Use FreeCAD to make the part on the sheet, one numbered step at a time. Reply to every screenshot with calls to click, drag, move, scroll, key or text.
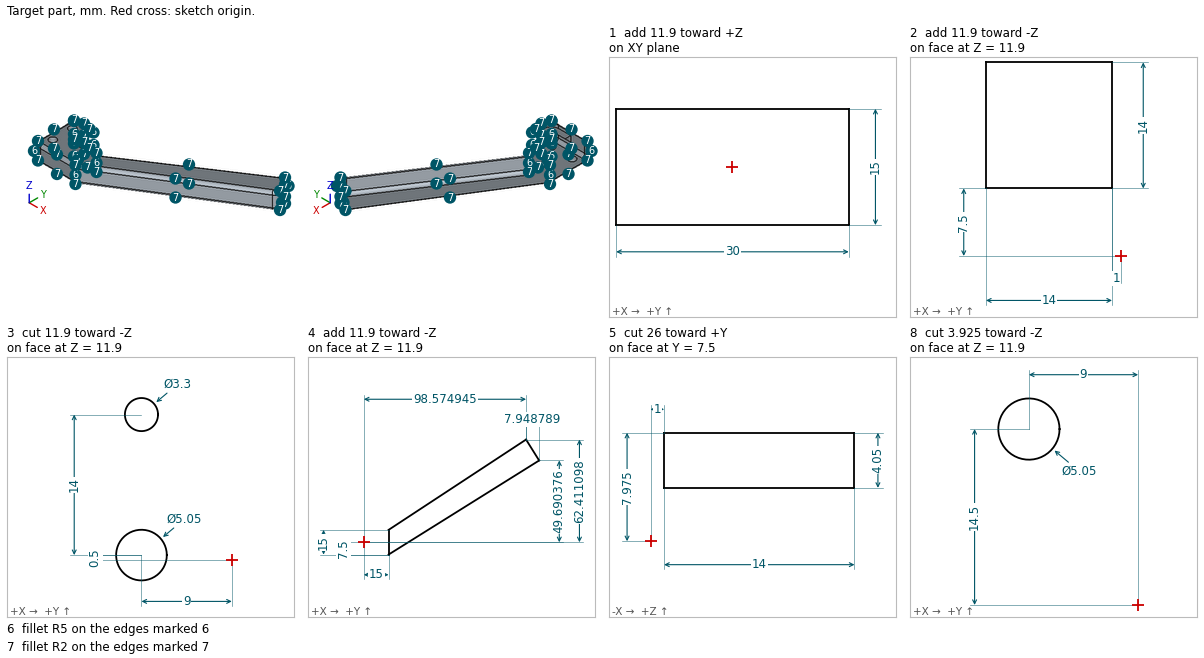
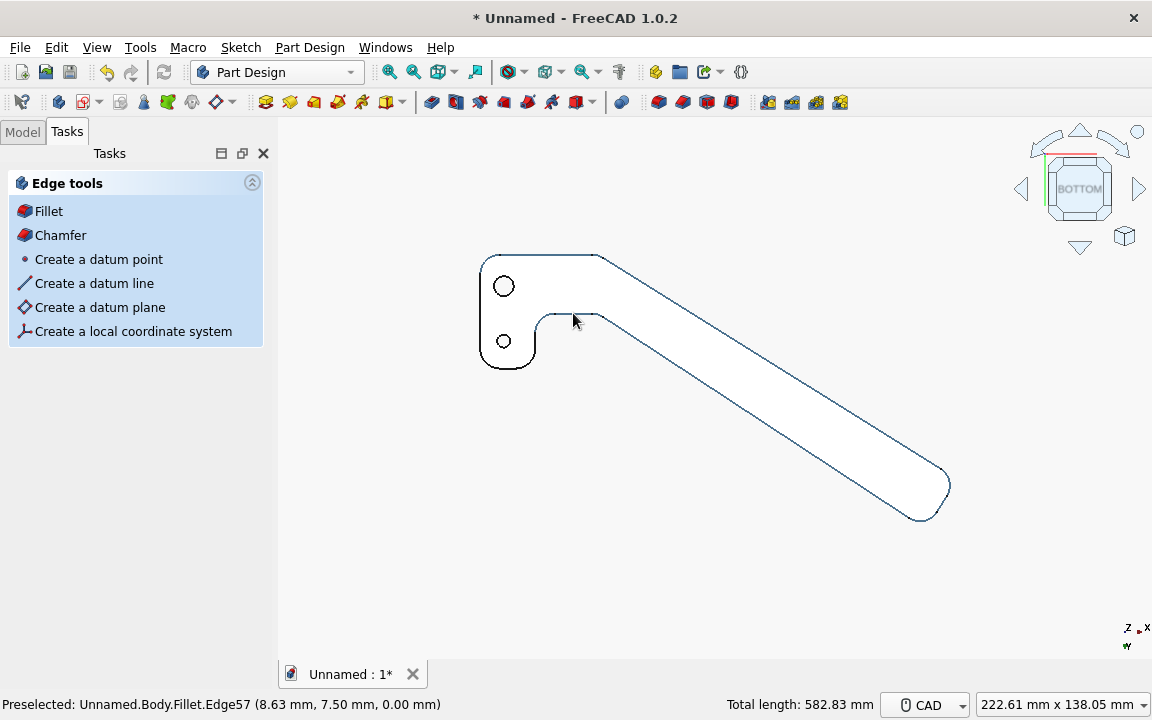
click(480, 349, ctrl)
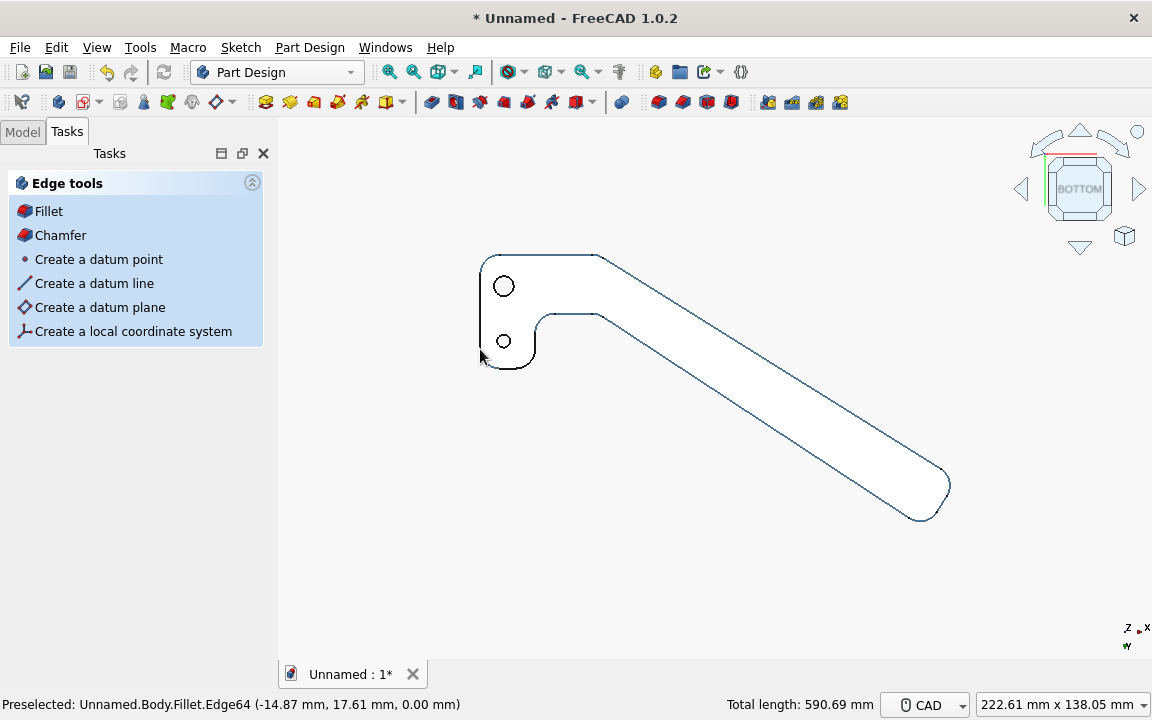
click(522, 367, ctrl)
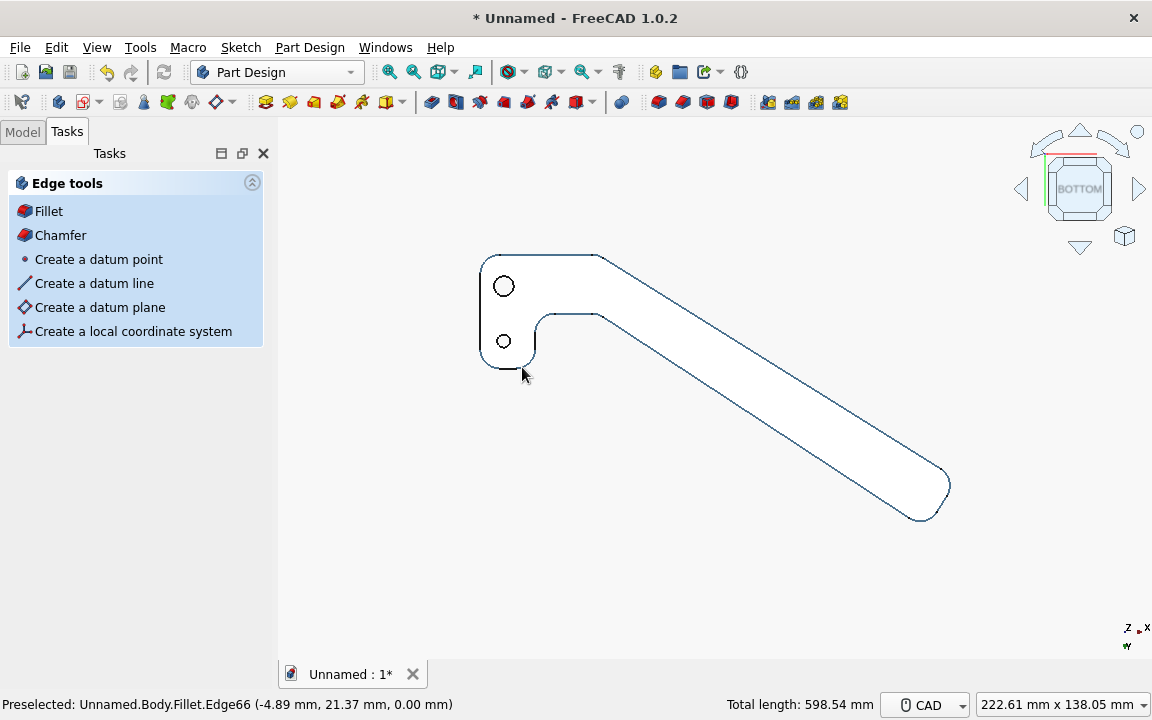
key(4)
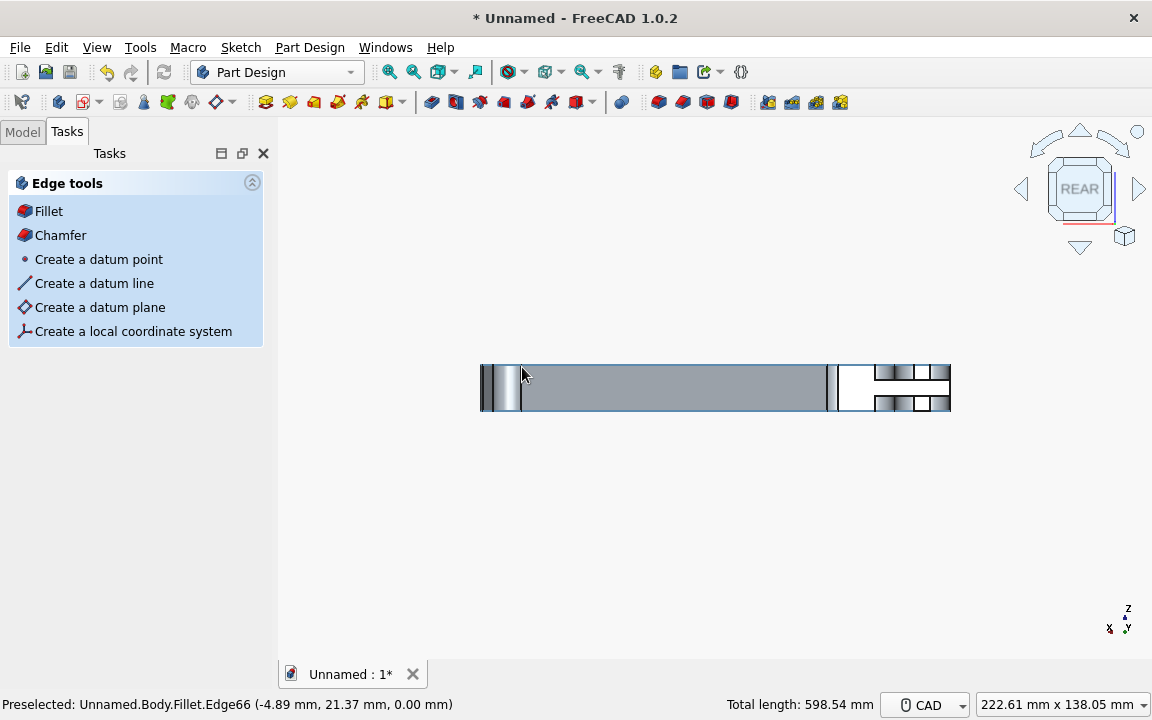
click(922, 410, ctrl)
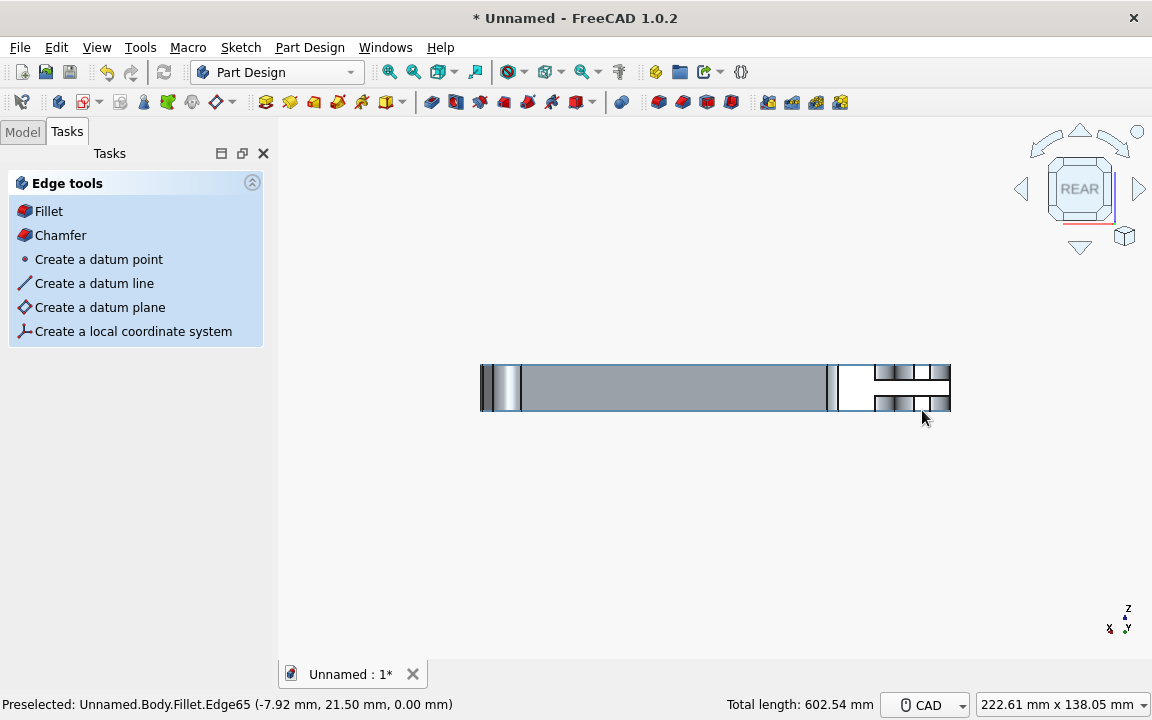
key(6)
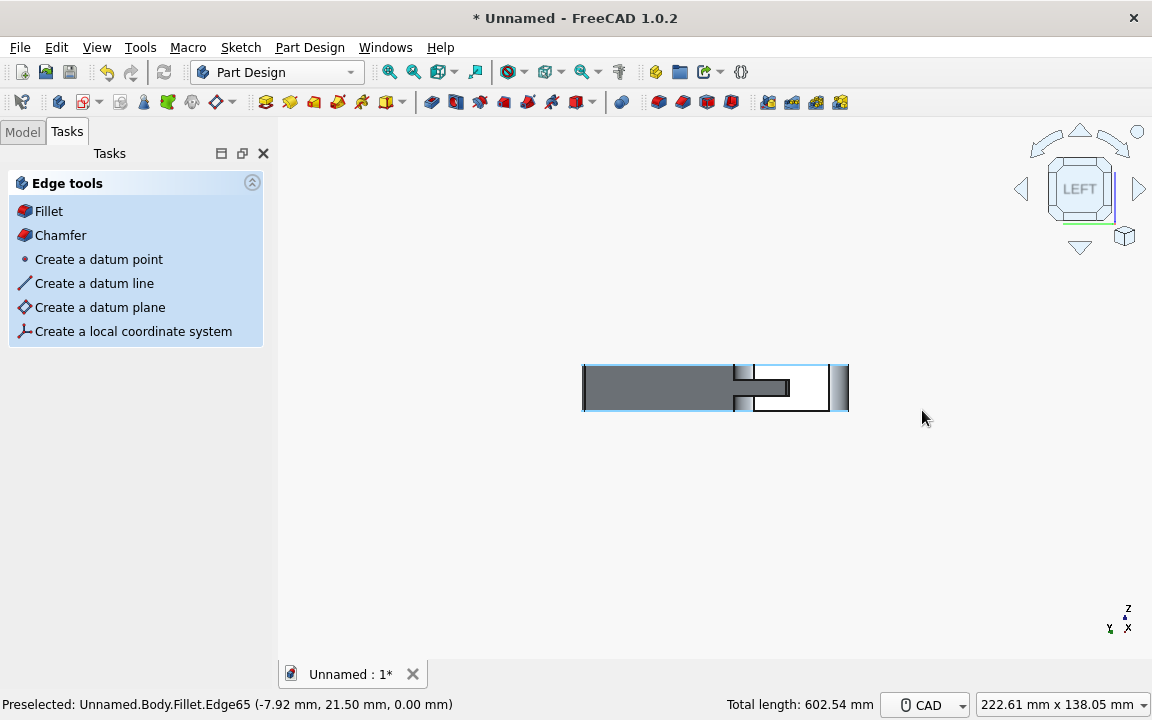
key(v)
key(f)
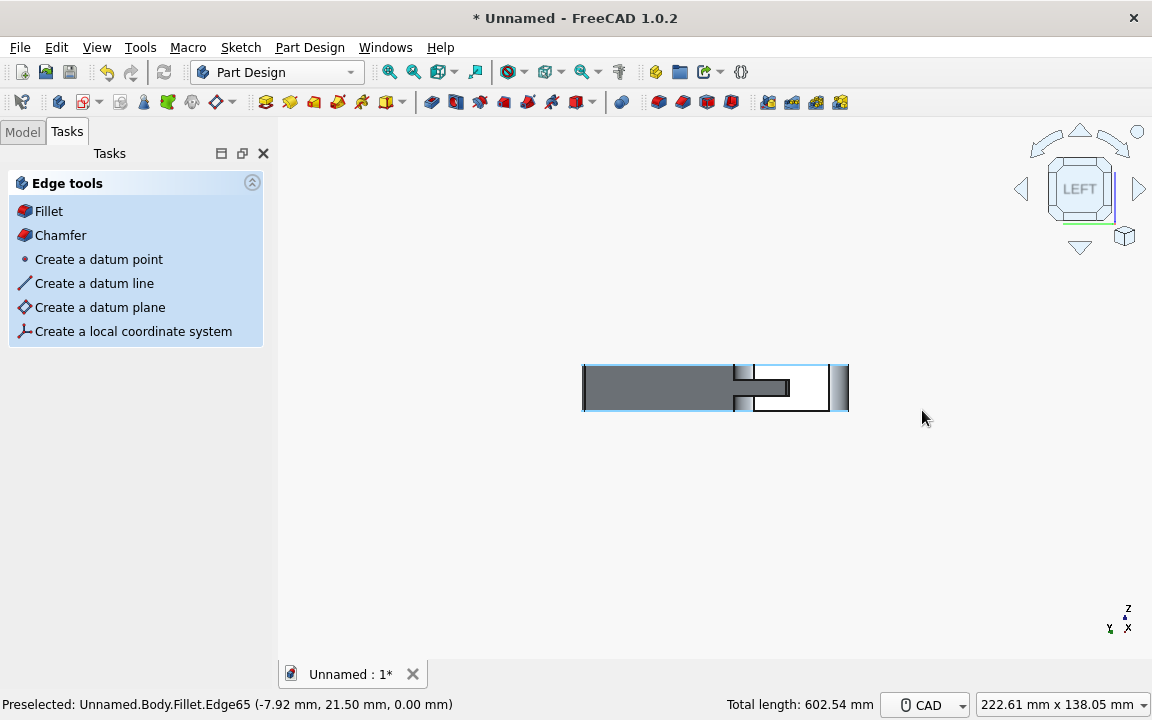
click(791, 410, ctrl)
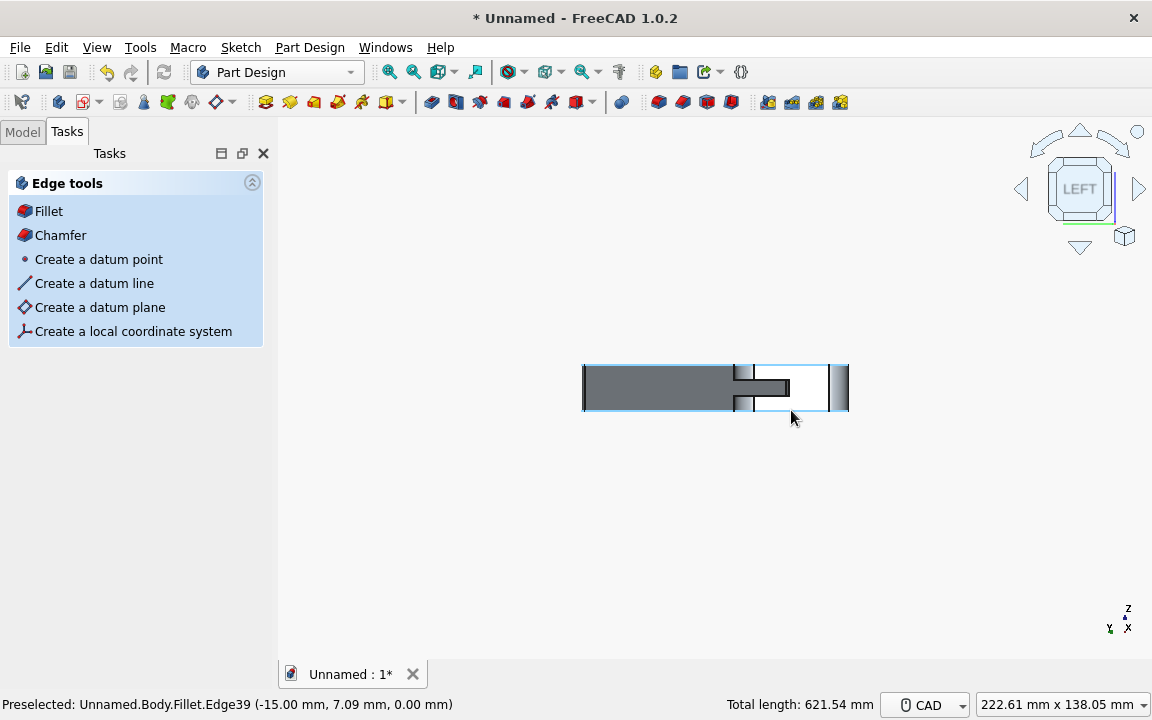
scroll(762, 410, up, 5)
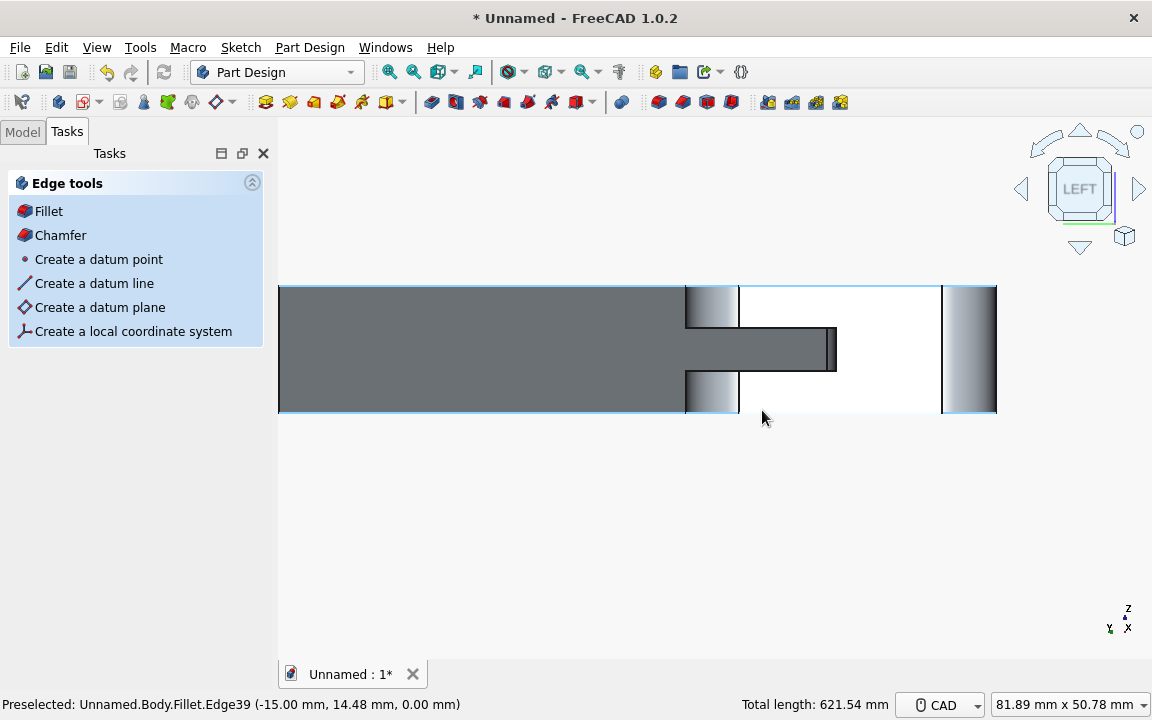
click(390, 72)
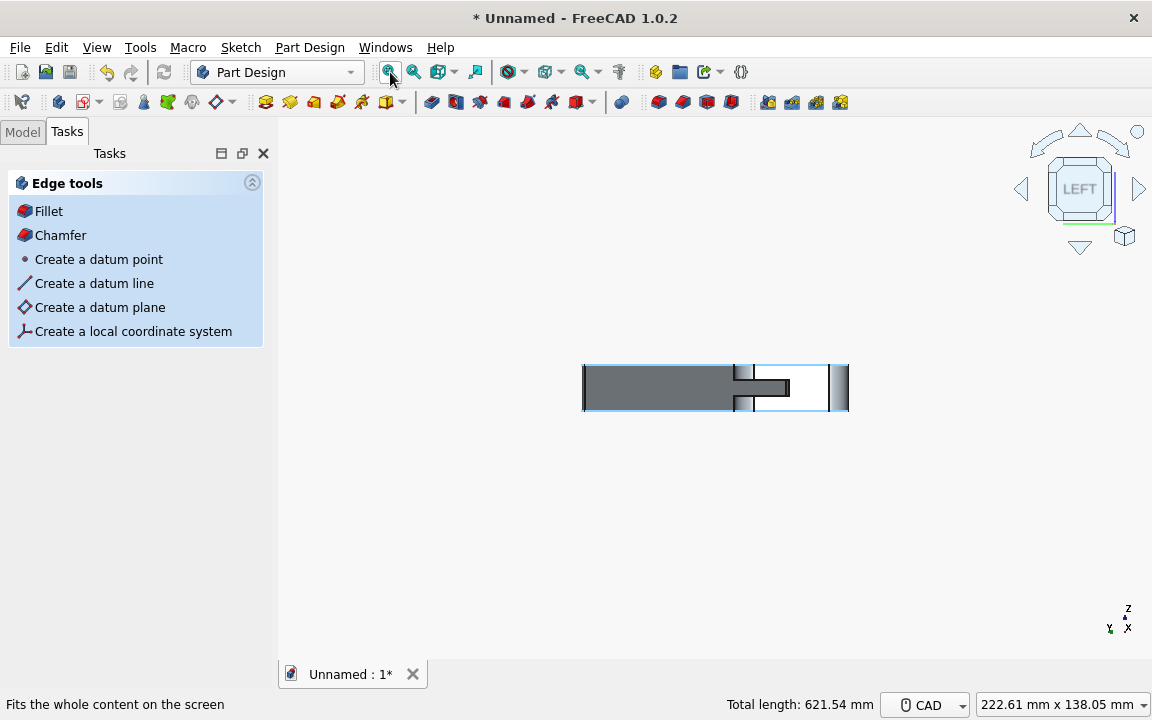
key(v)
key(3)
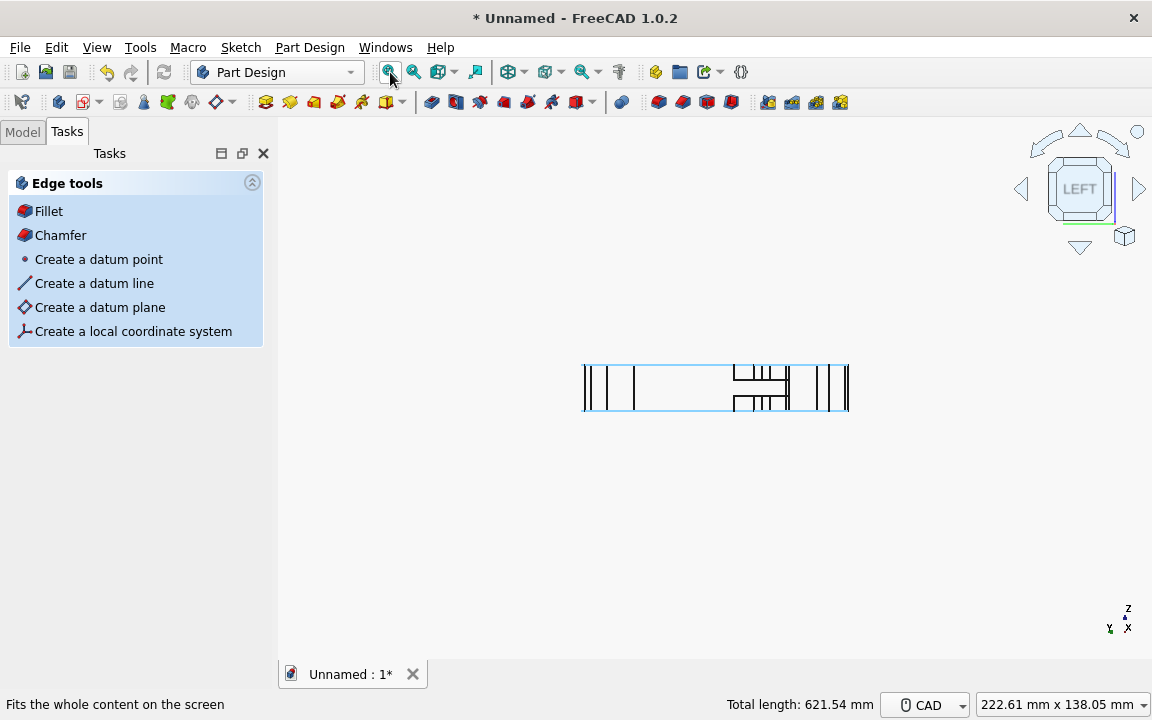
key(0)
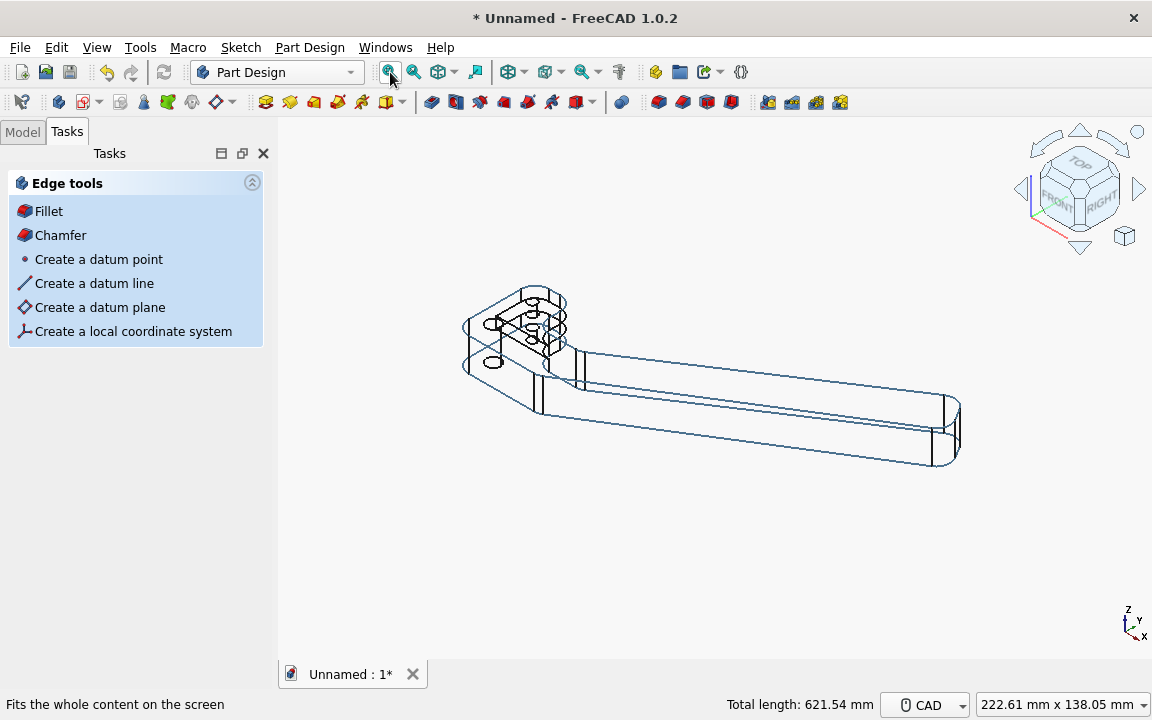
click(556, 351, ctrl)